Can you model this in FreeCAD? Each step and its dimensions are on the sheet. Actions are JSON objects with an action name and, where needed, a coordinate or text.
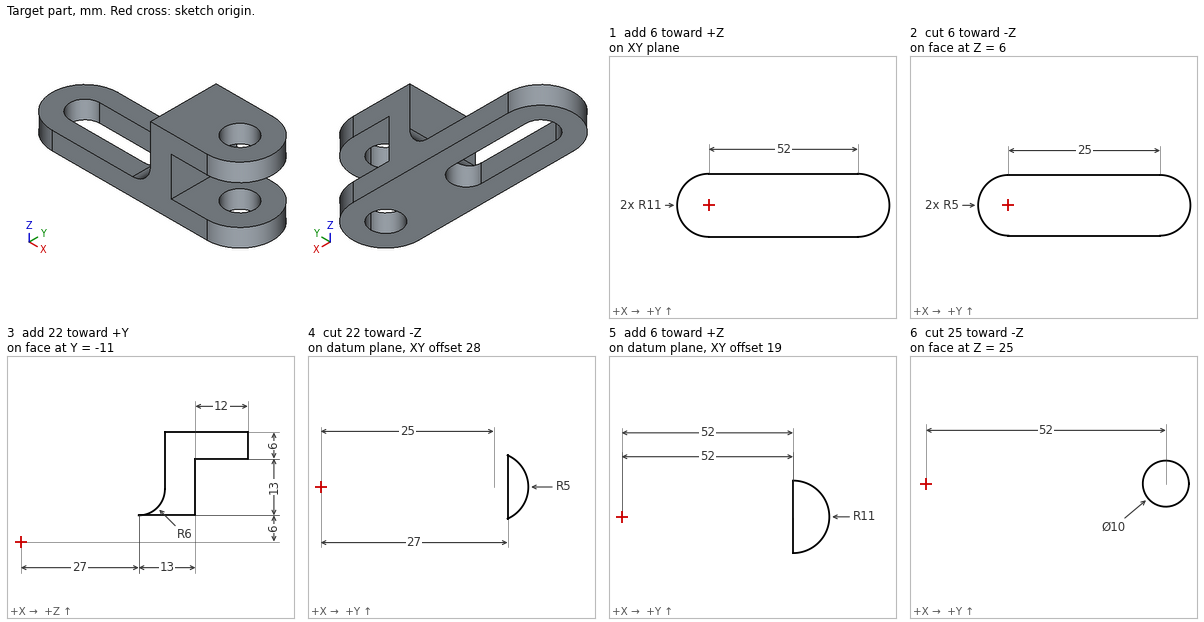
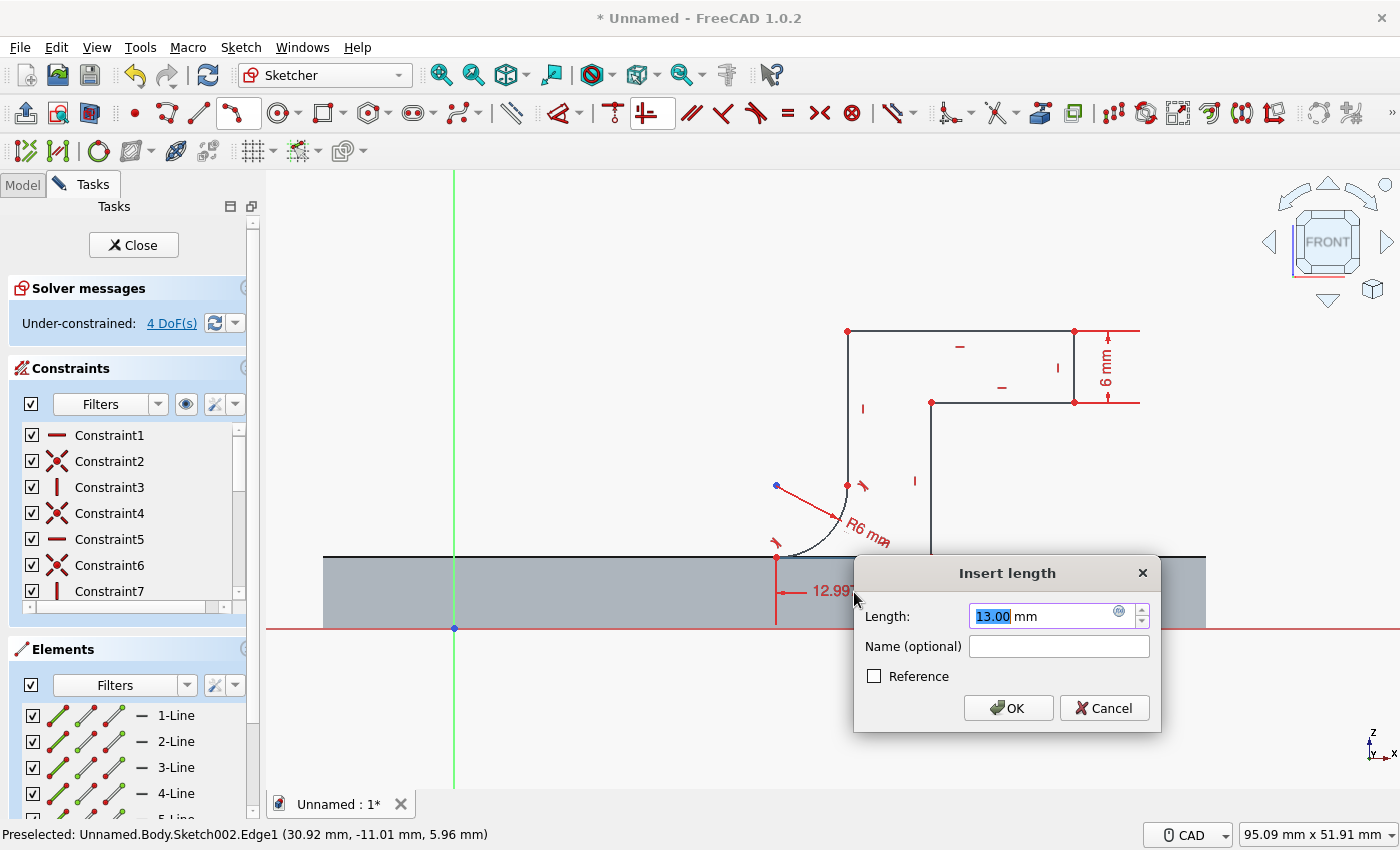
{"action": "type", "text": "13"}
{"action": "key", "text": "Return"}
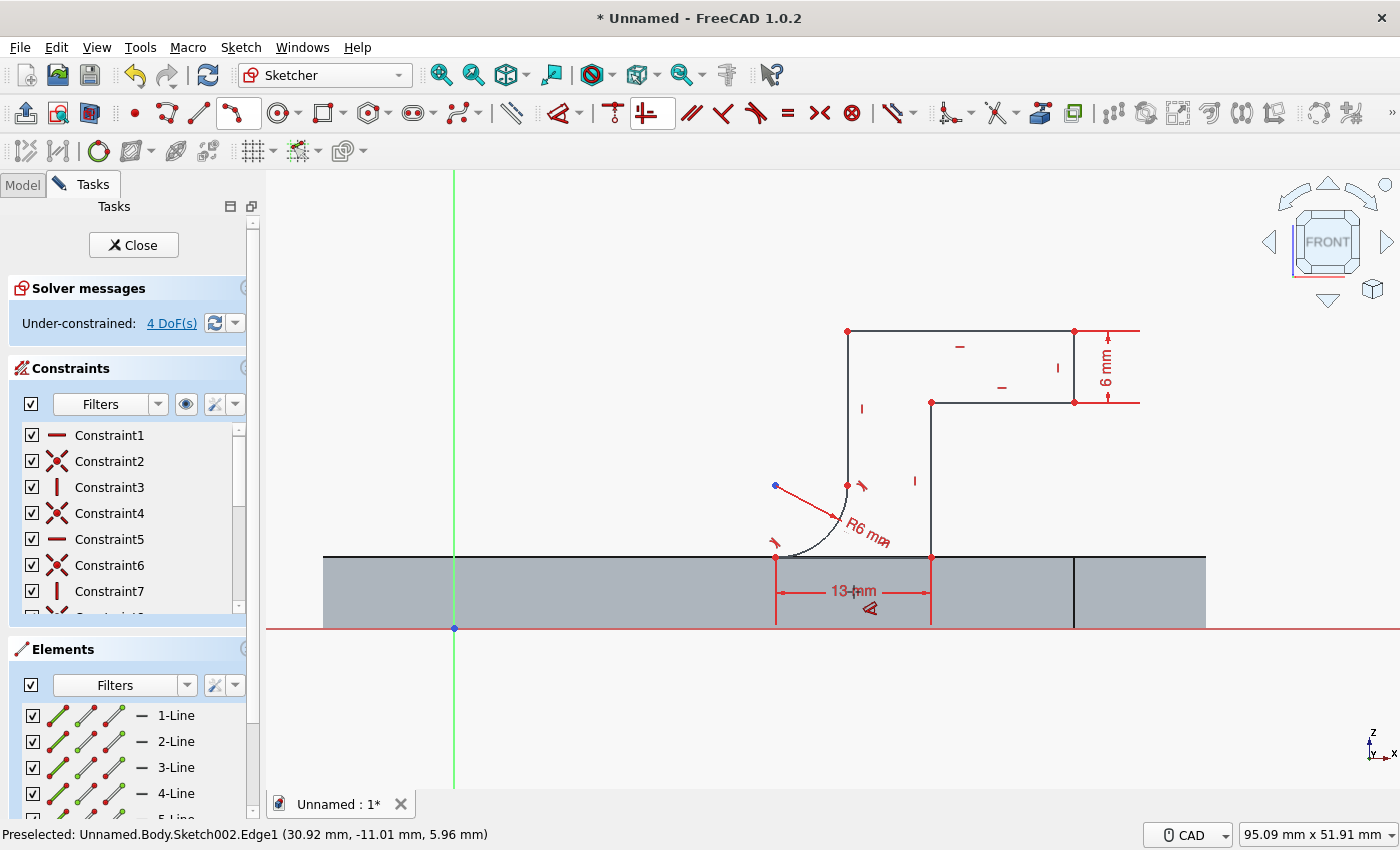
{"action": "left_click", "coordinate": [931, 511]}
{"action": "left_click", "coordinate": [965, 480]}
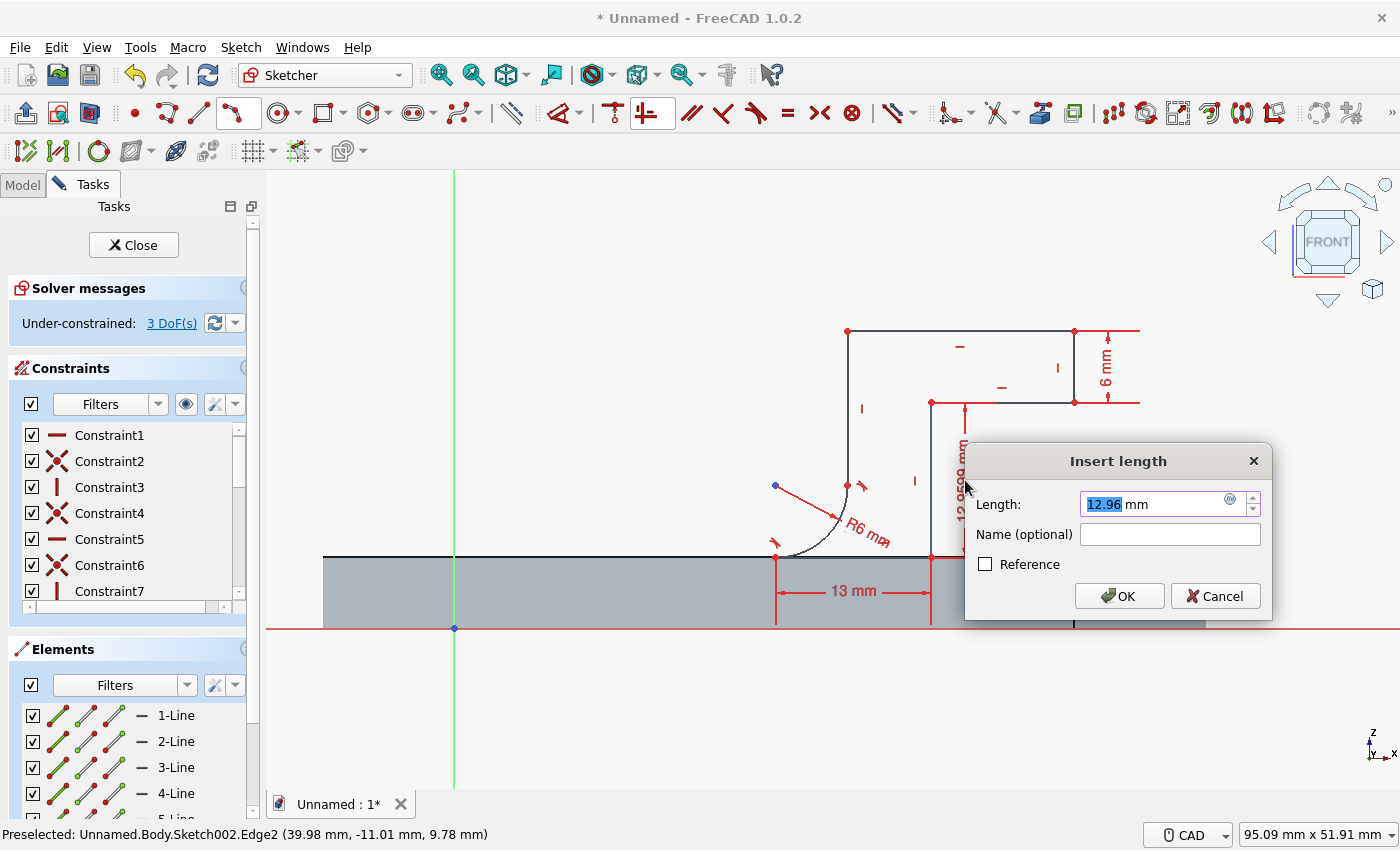
{"action": "type", "text": "13"}
{"action": "key", "text": "Return"}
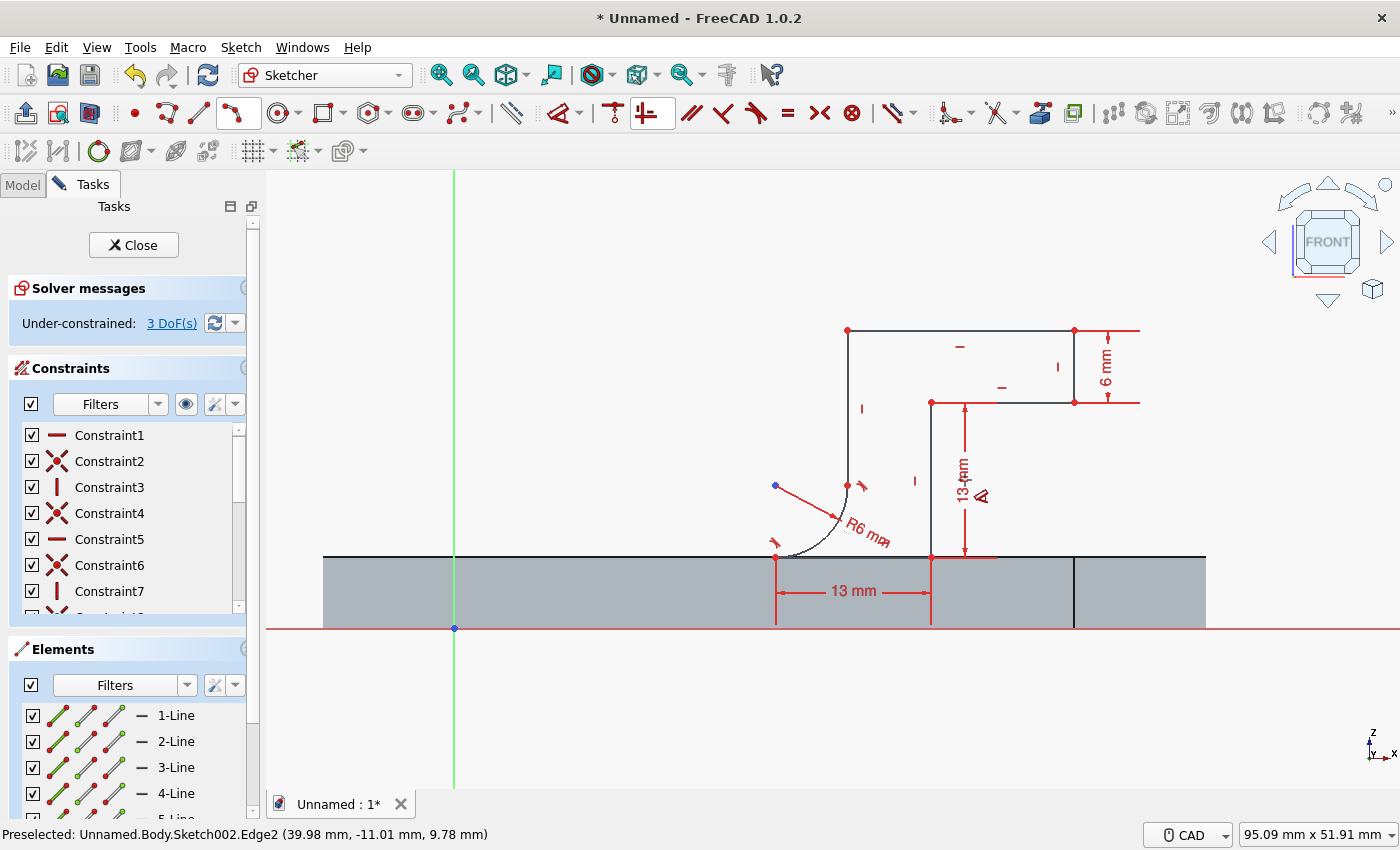
{"action": "left_click", "coordinate": [974, 403]}
{"action": "left_click", "coordinate": [1002, 369]}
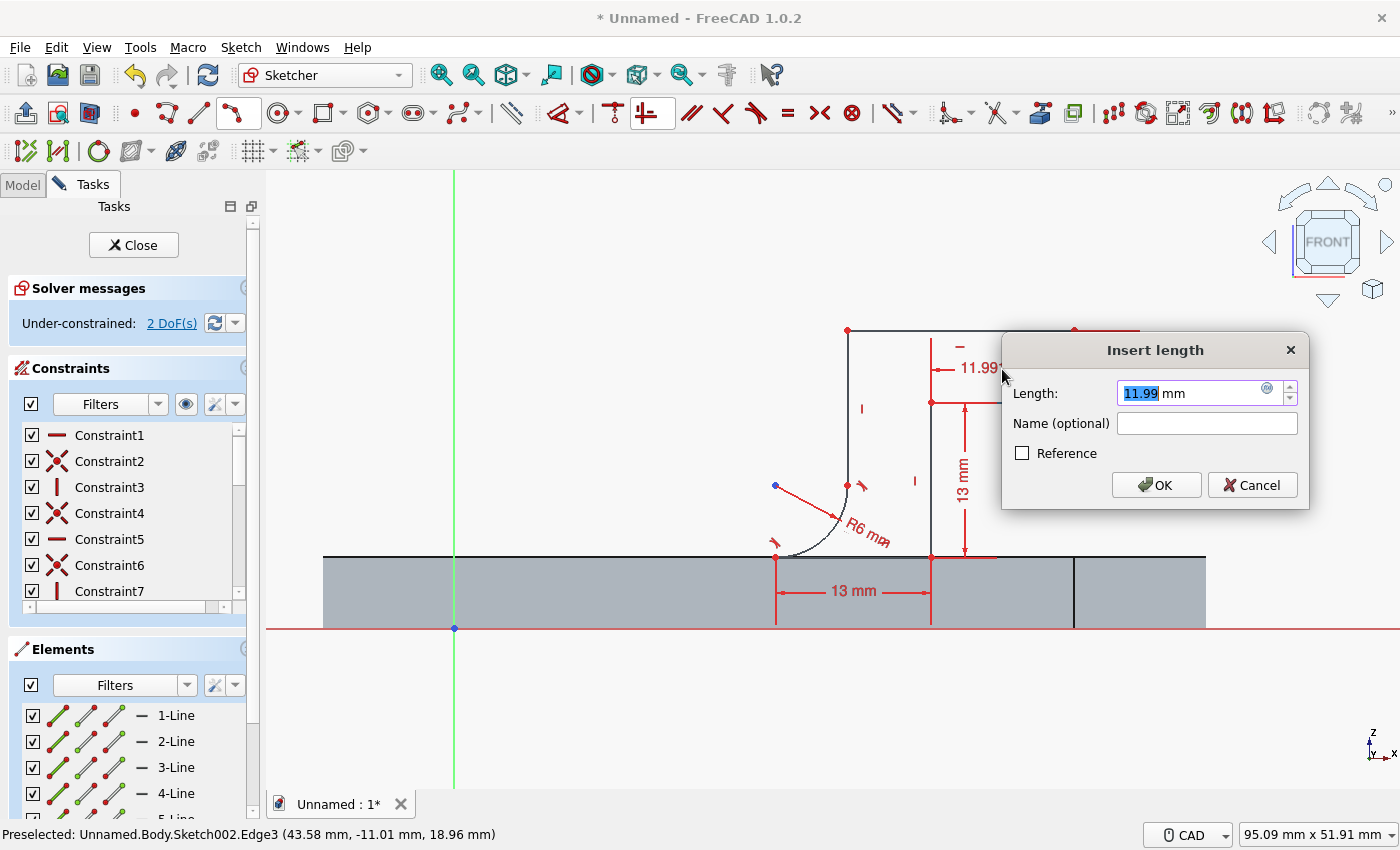
{"action": "type", "text": "12"}
{"action": "key", "text": "Return"}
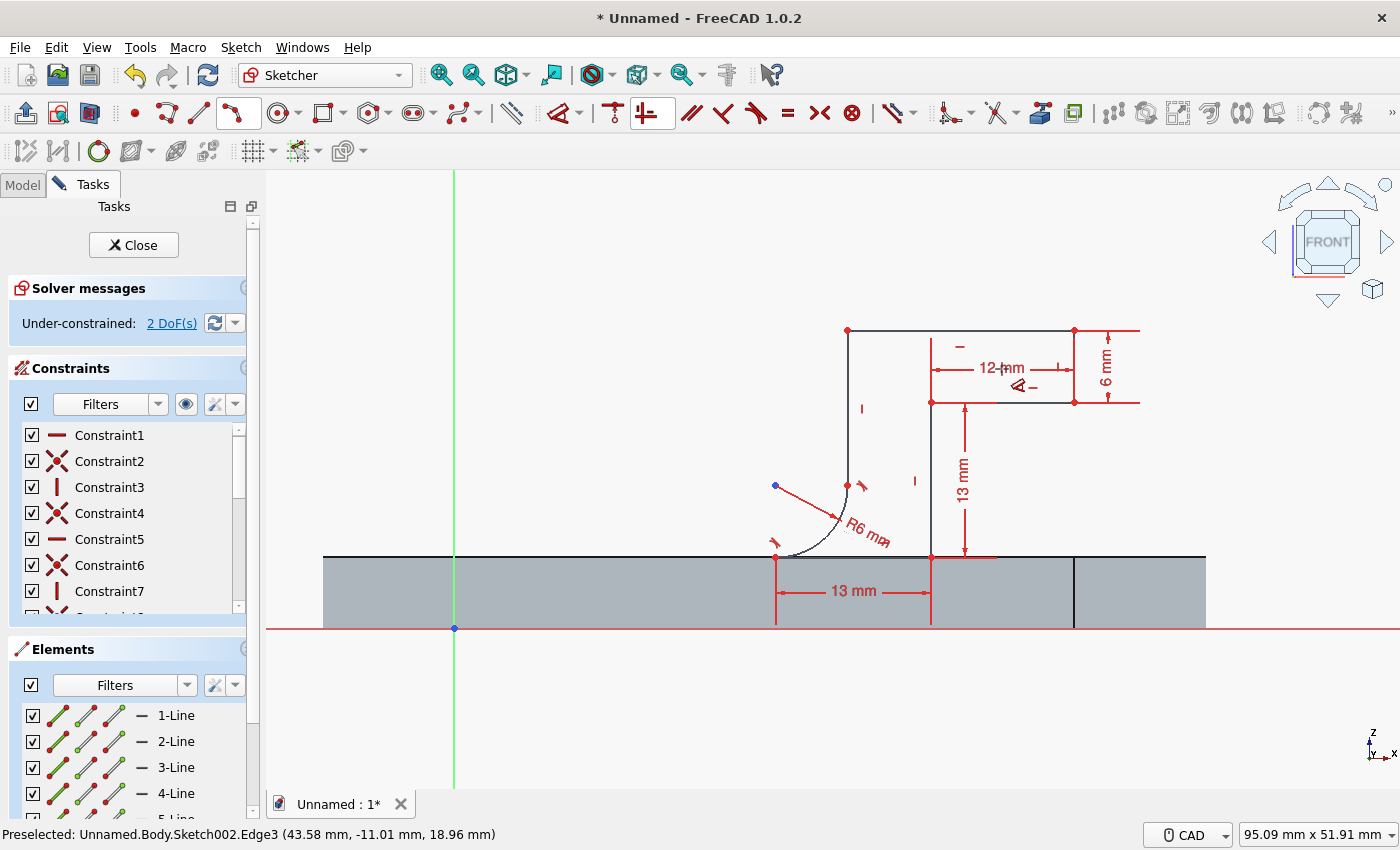
{"action": "left_click", "coordinate": [776, 558]}
{"action": "left_click", "coordinate": [420, 593]}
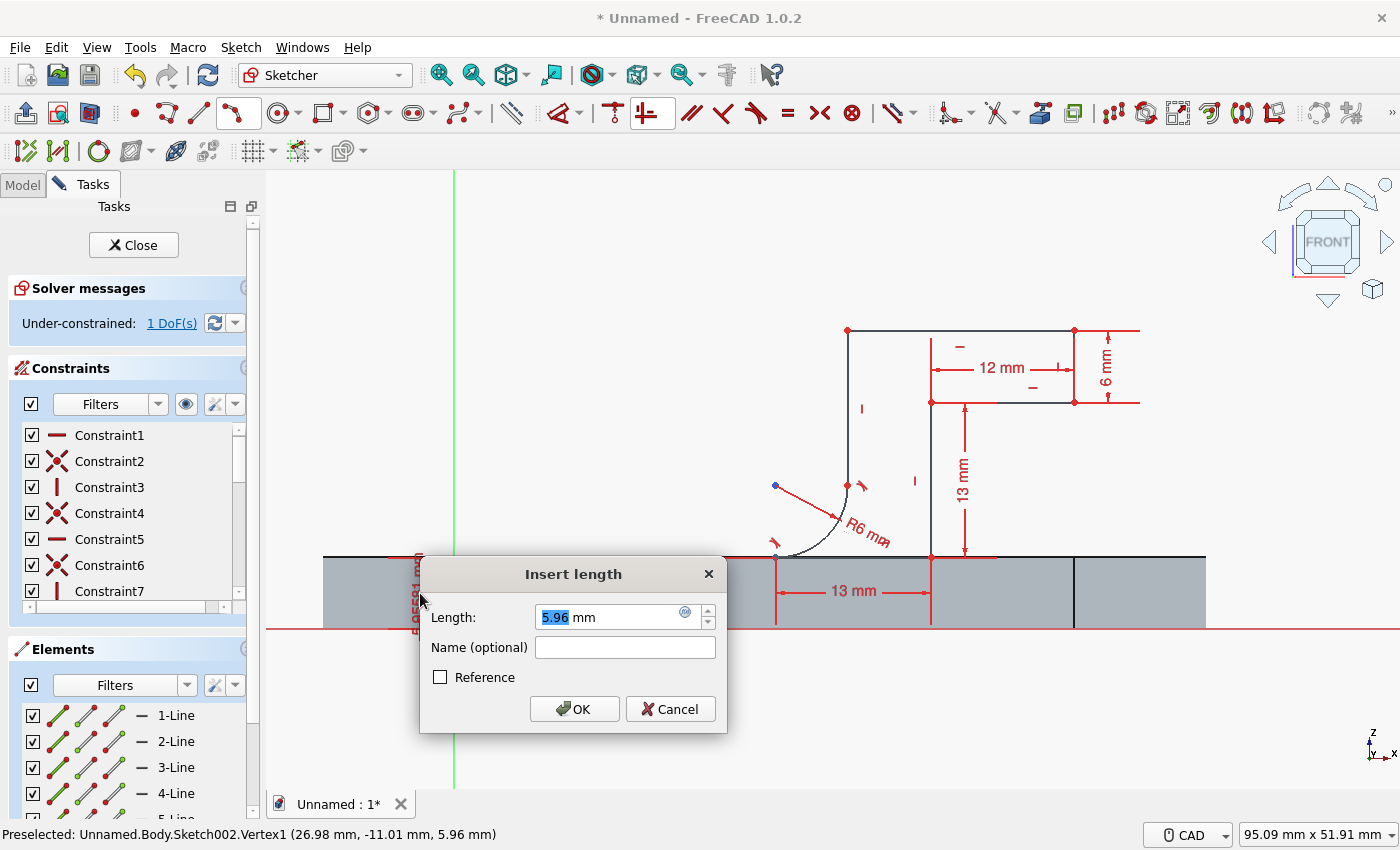
{"action": "type", "text": "6"}
{"action": "key", "text": "Return"}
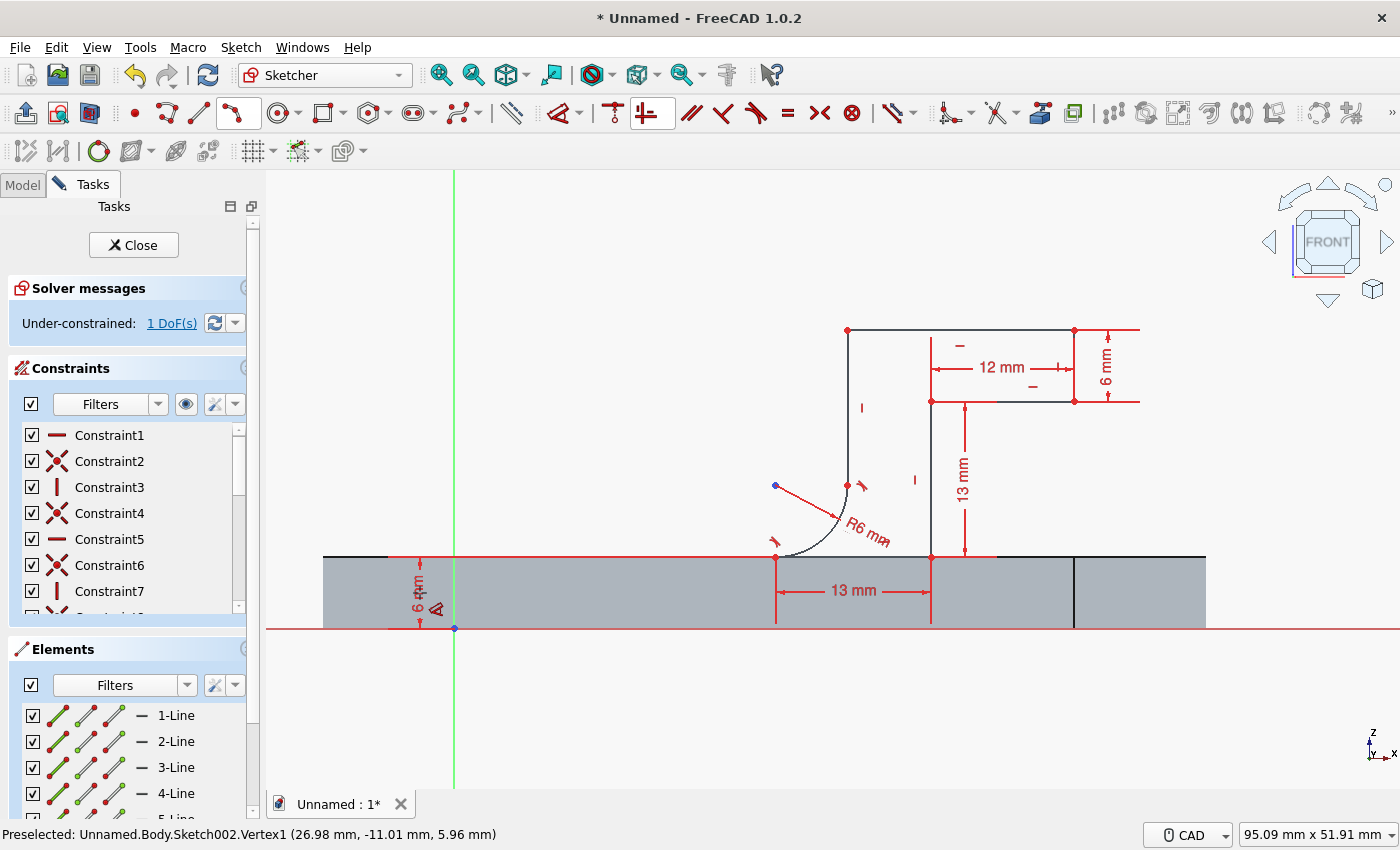
{"action": "left_click", "coordinate": [776, 557]}
{"action": "left_click", "coordinate": [615, 663]}